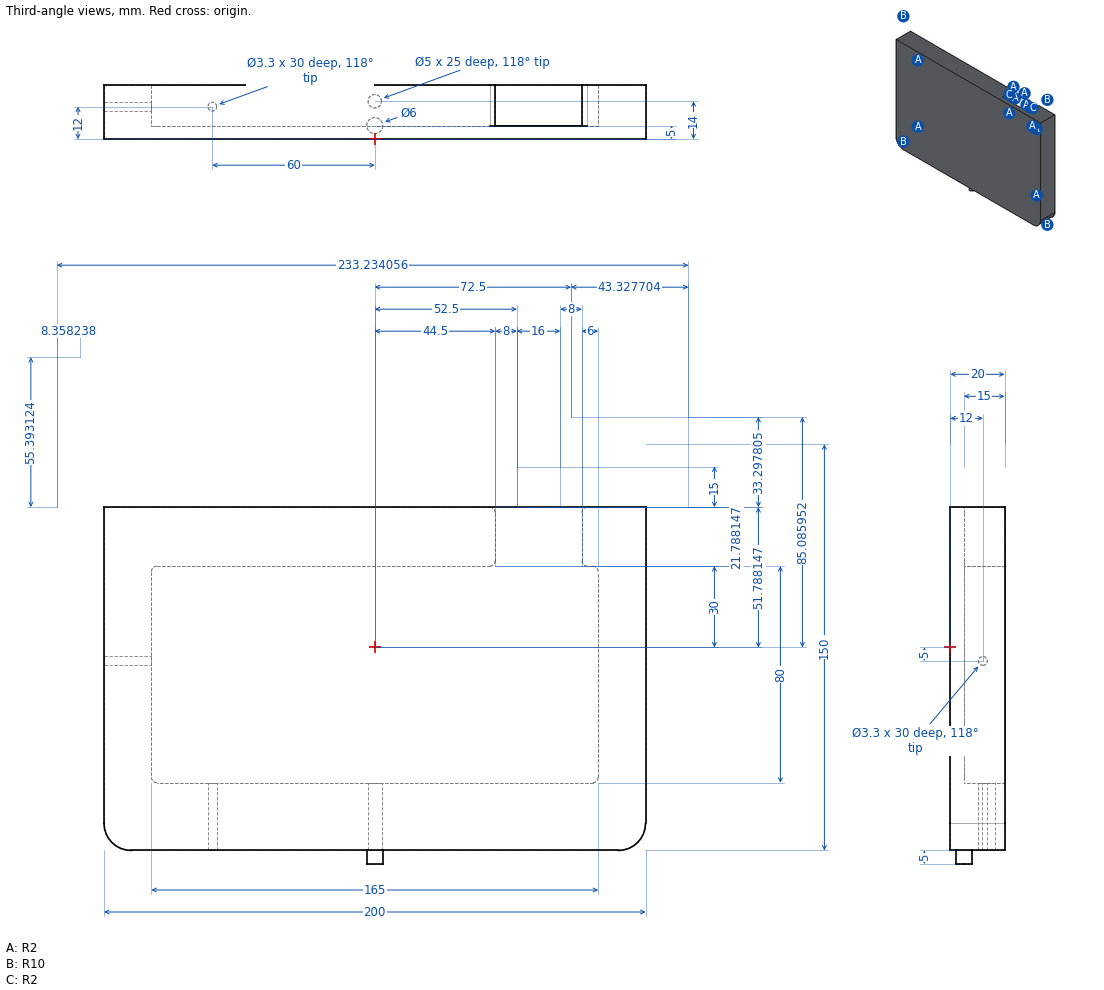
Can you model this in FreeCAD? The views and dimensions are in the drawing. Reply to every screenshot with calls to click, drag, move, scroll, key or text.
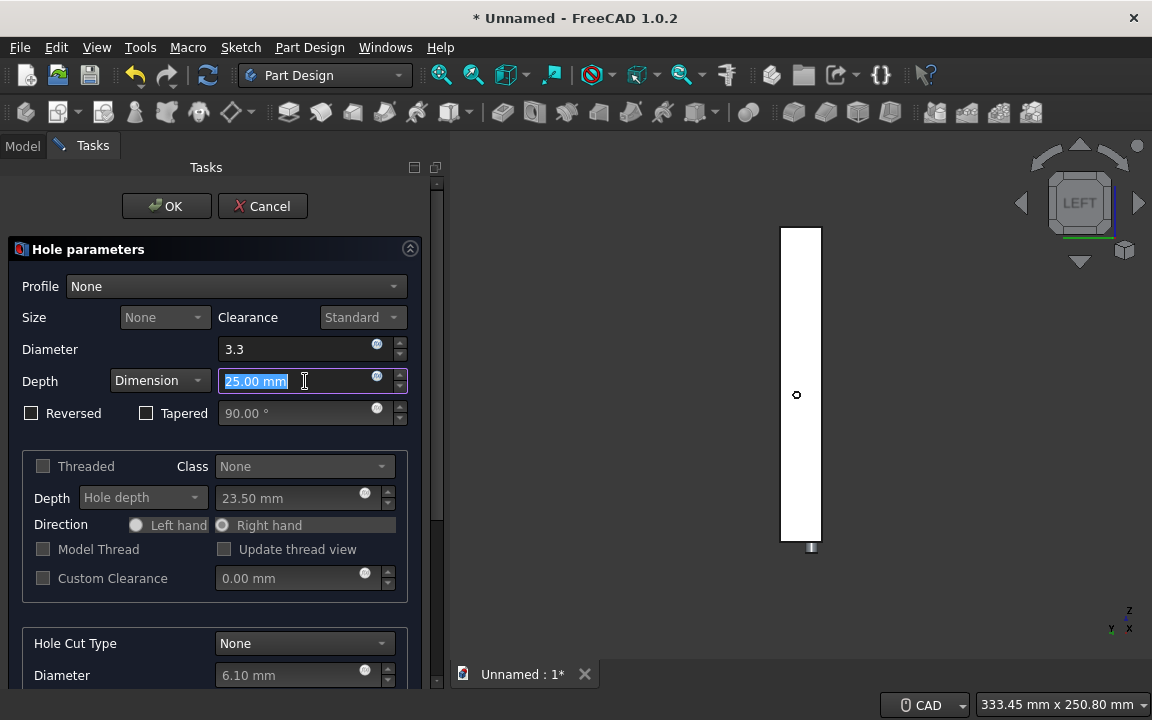
text(30)
key(Tab)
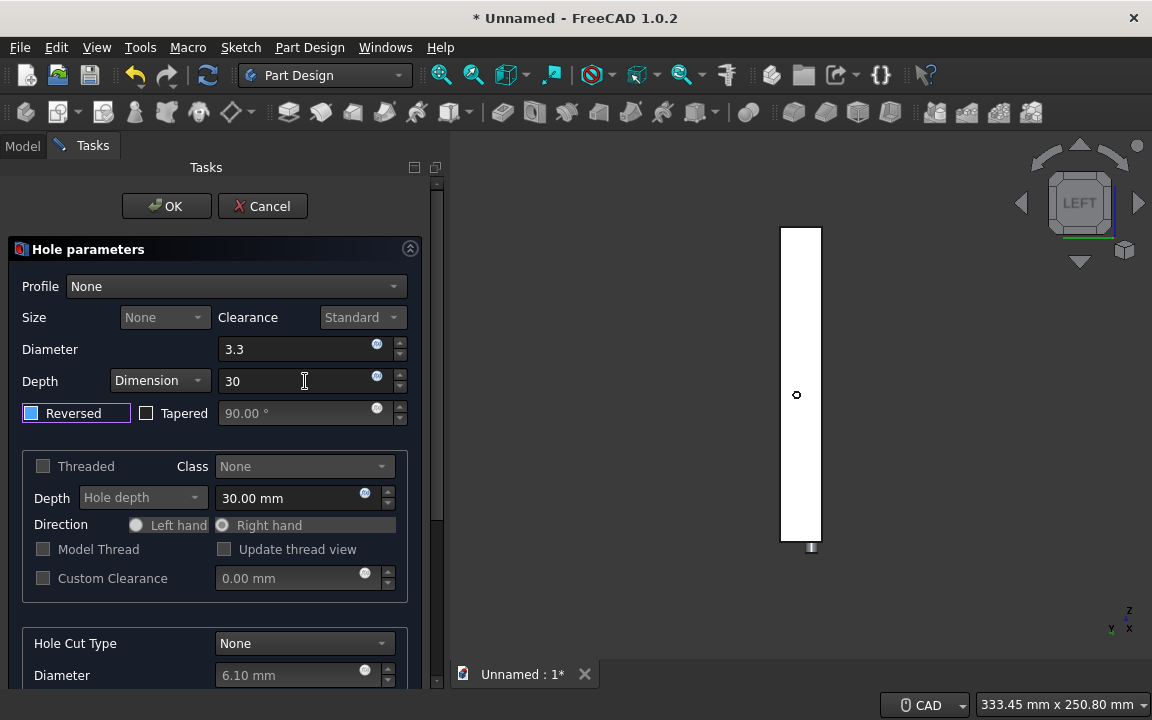
click(167, 206)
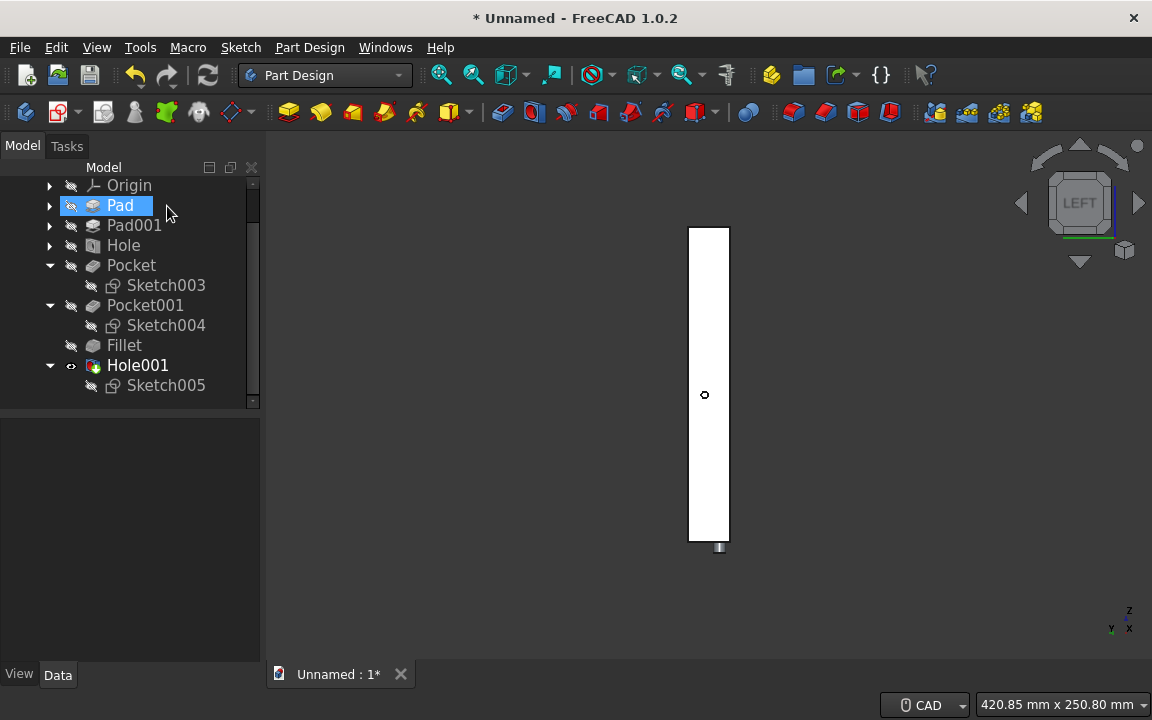
click(709, 226)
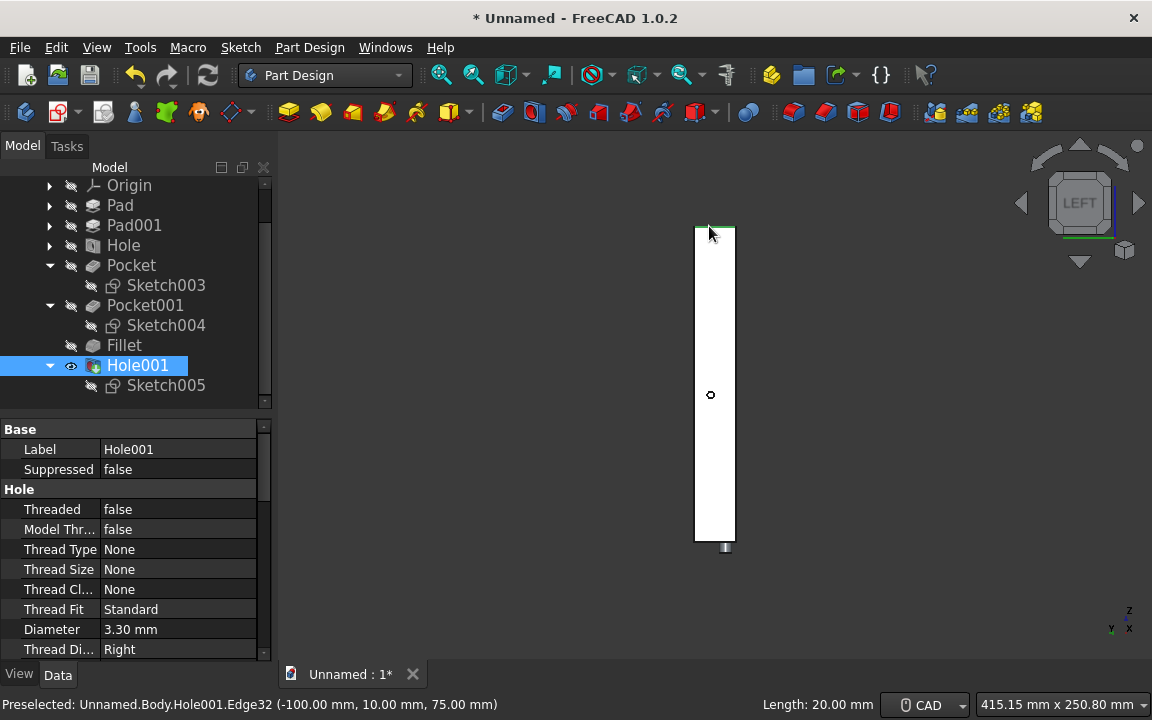
click(715, 541, ctrl)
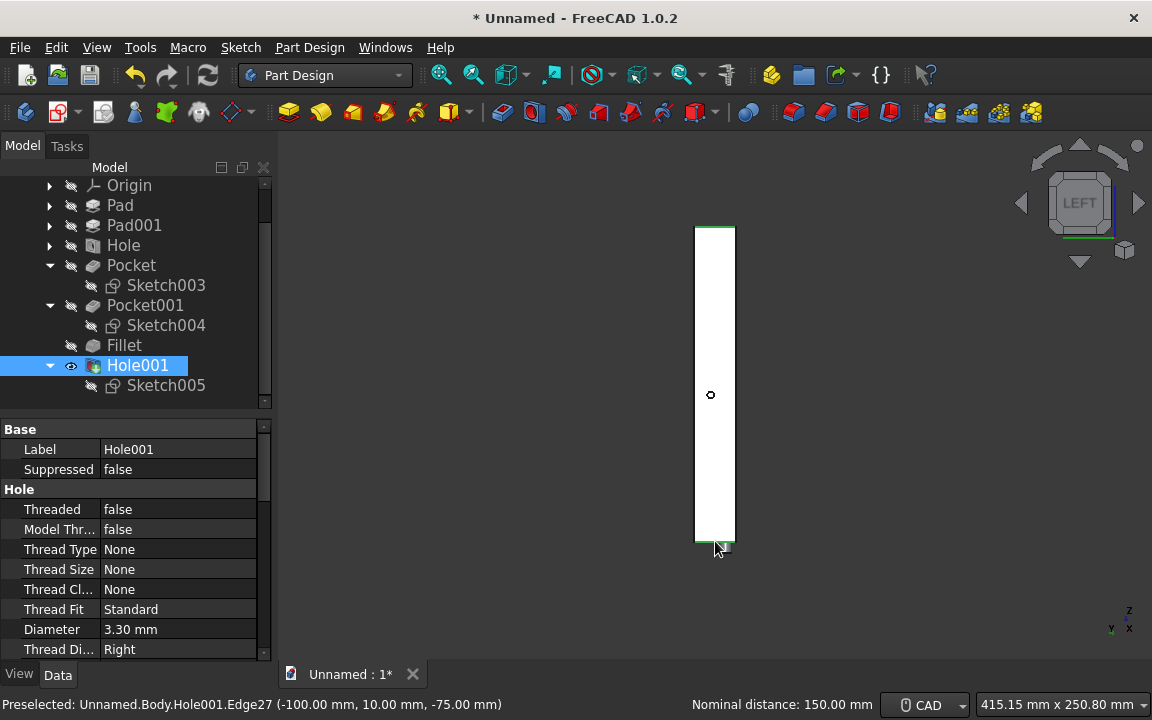
key(0)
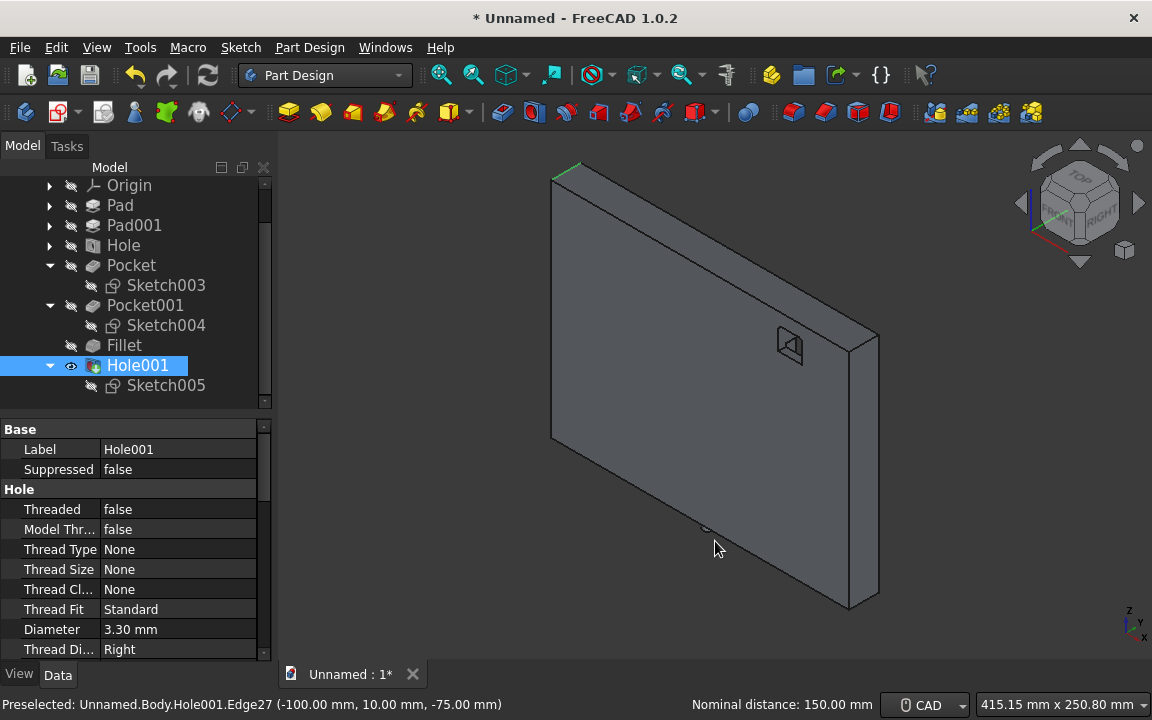
click(864, 342, ctrl)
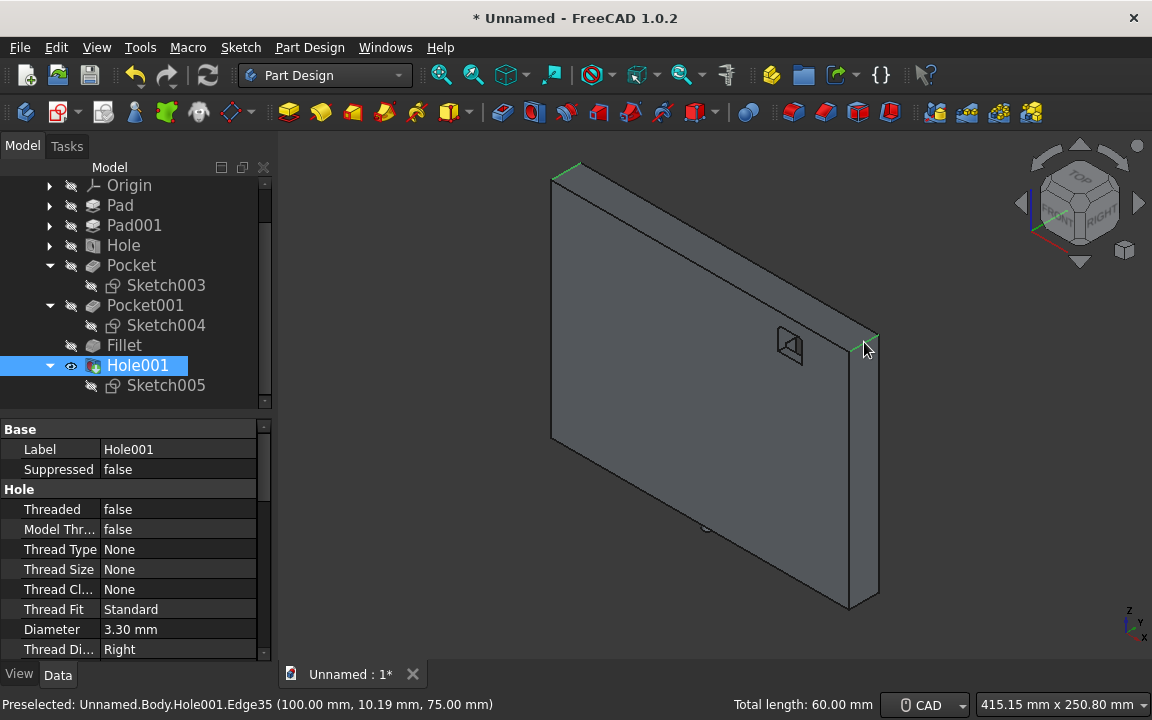
key(2)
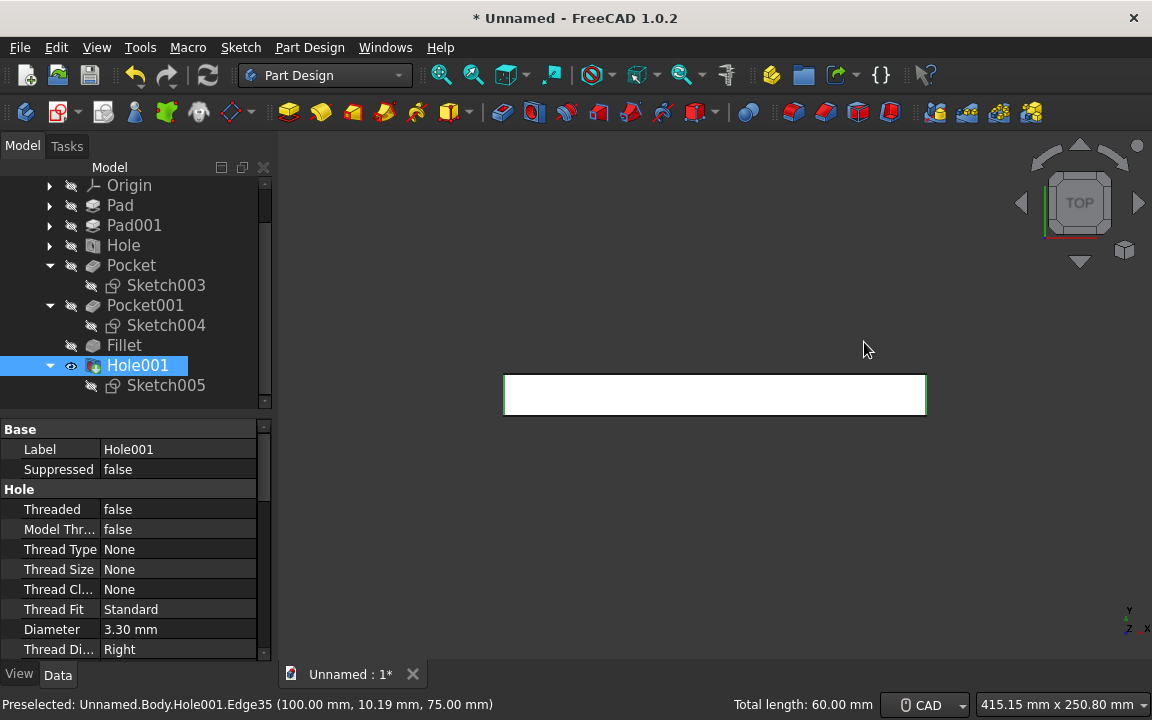
key(1)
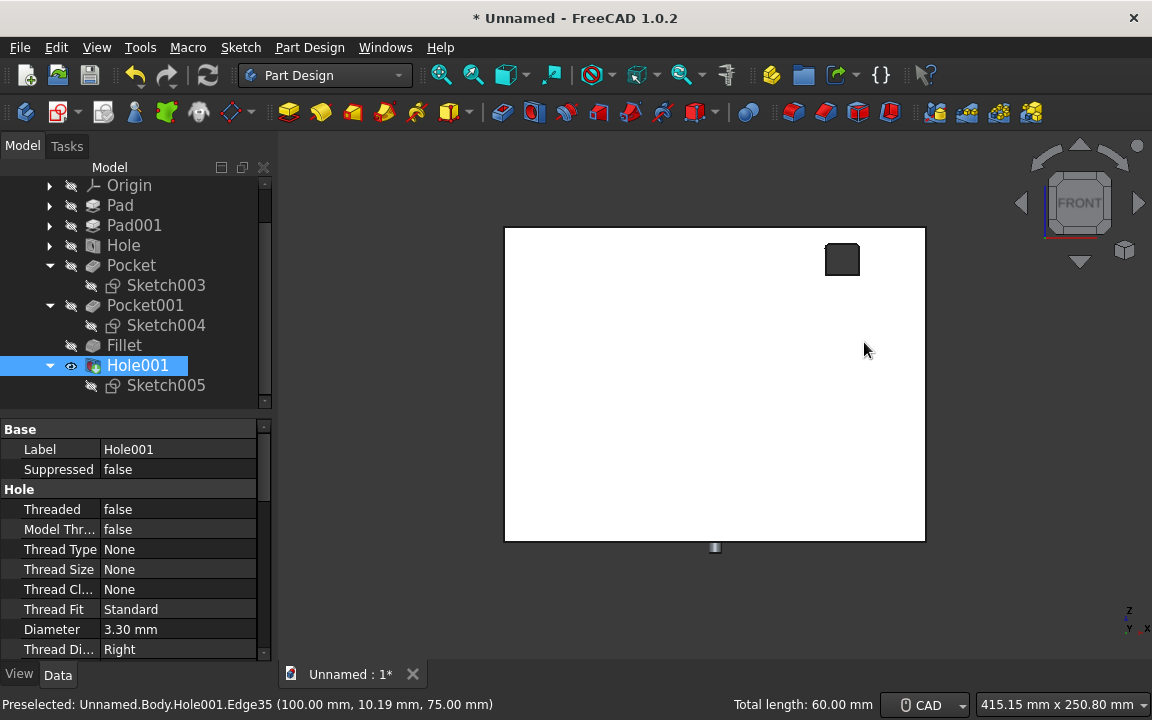
key(3)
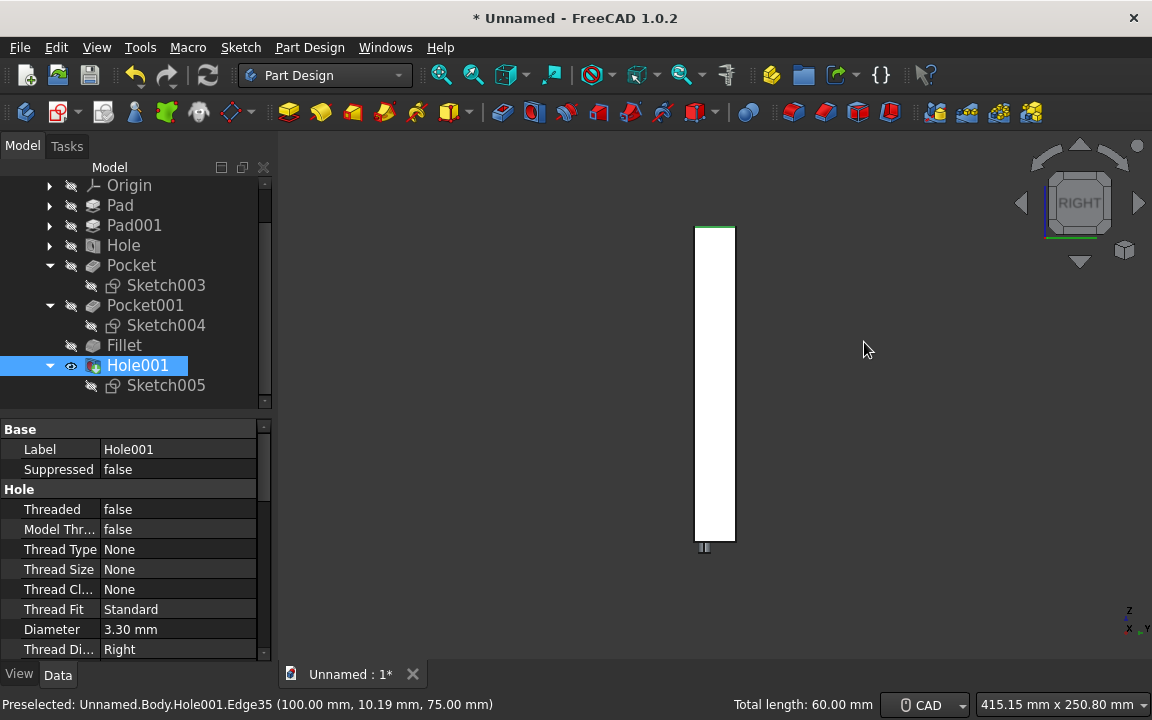
click(715, 541, ctrl)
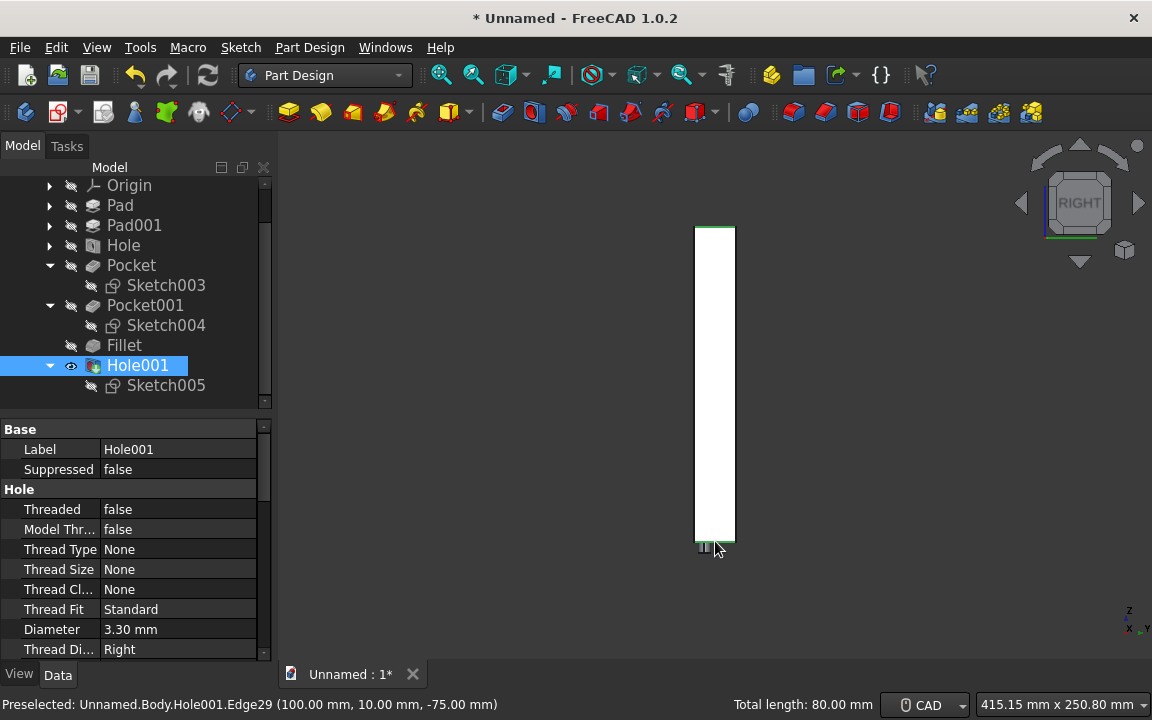
click(794, 112)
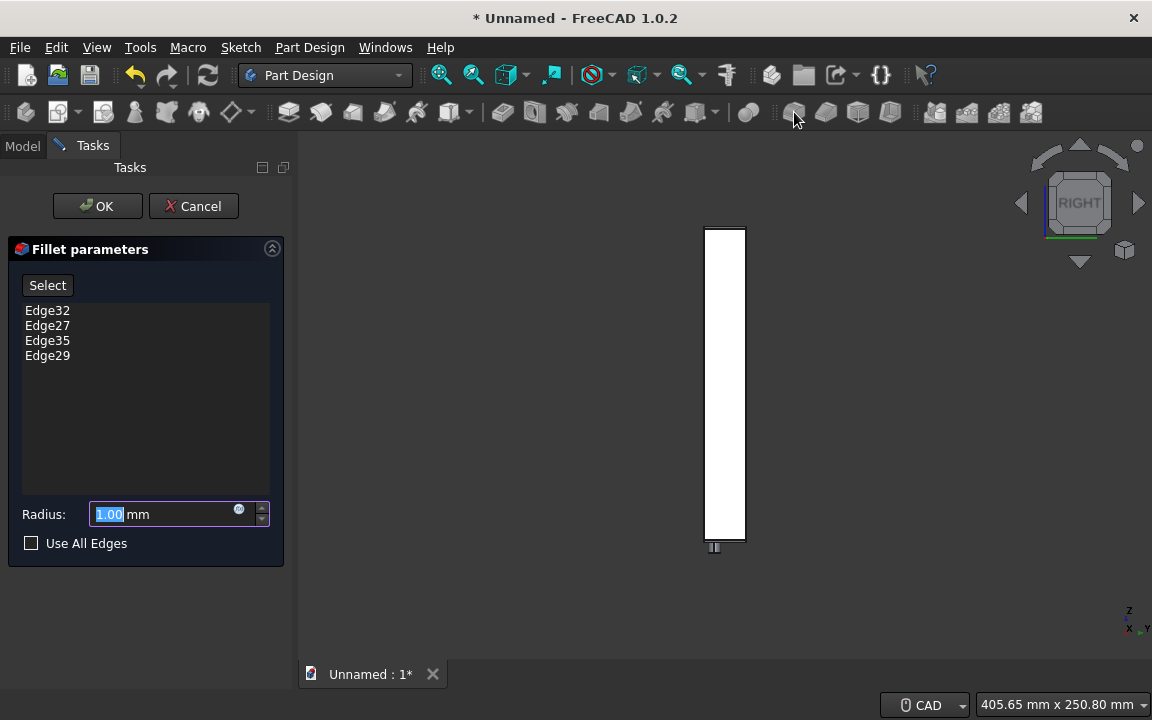
text(10)
key(Tab)